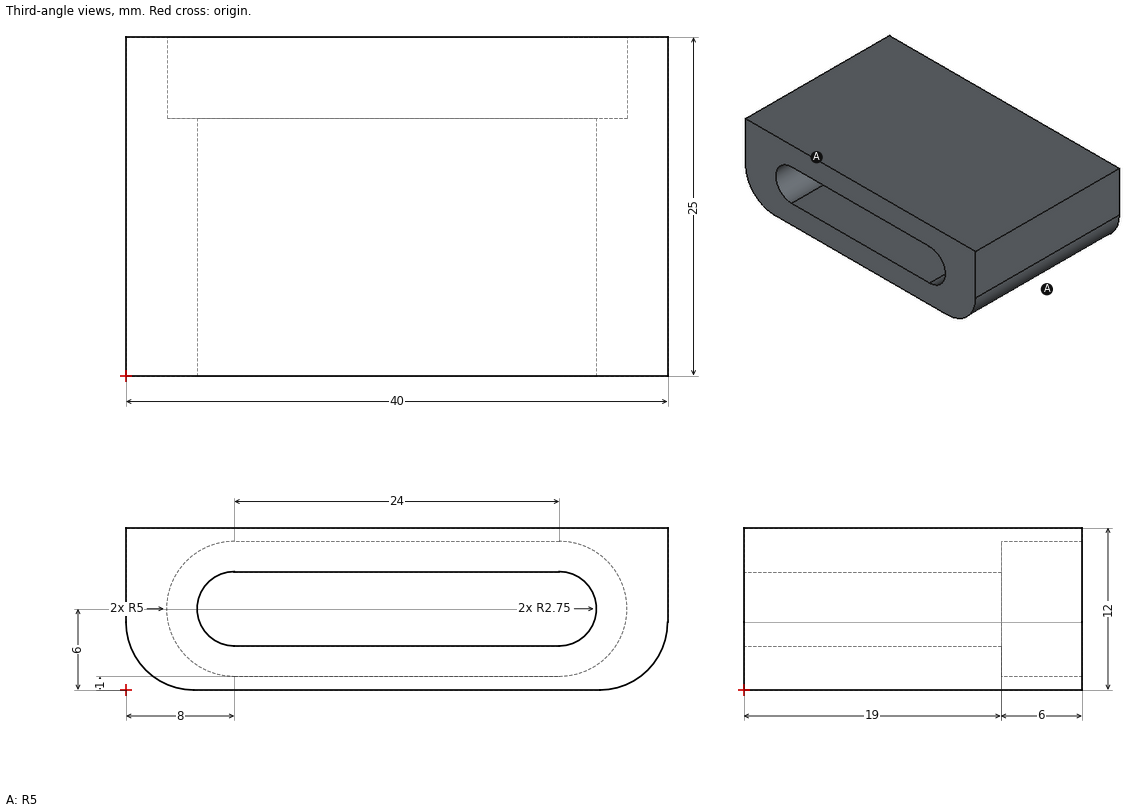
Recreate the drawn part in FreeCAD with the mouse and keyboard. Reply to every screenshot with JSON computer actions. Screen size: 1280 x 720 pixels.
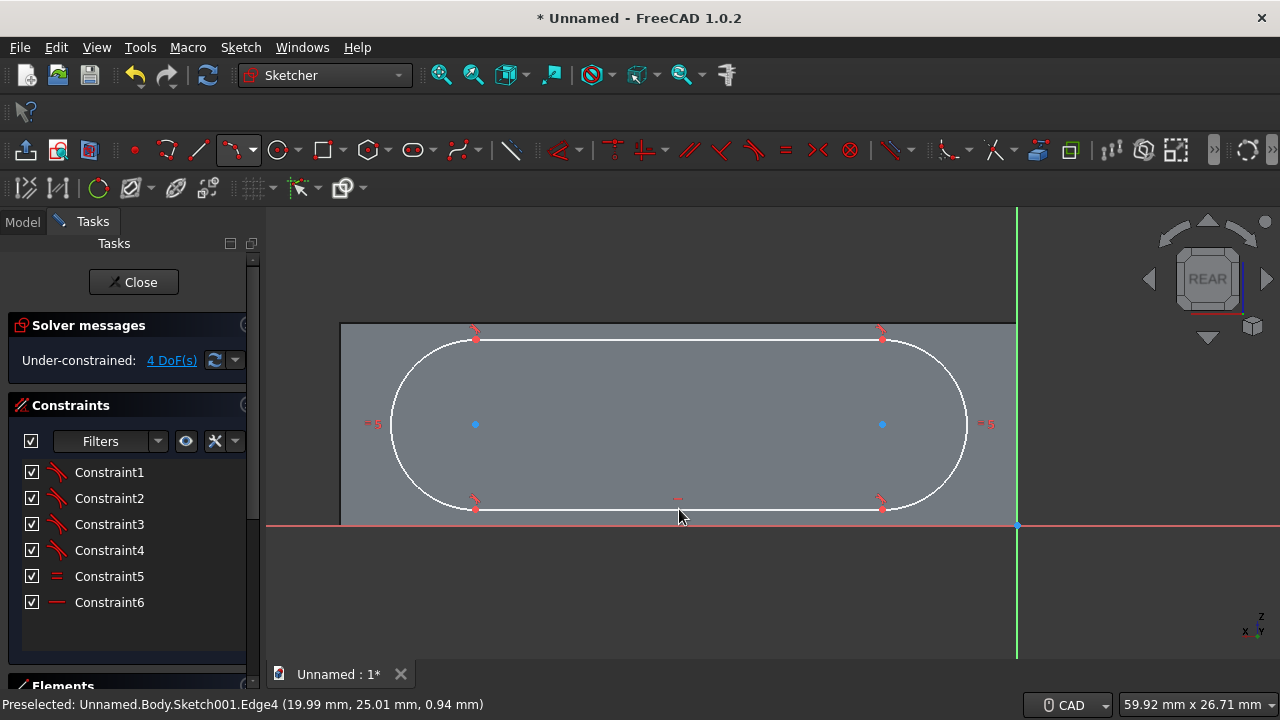
{"action": "key", "text": "d"}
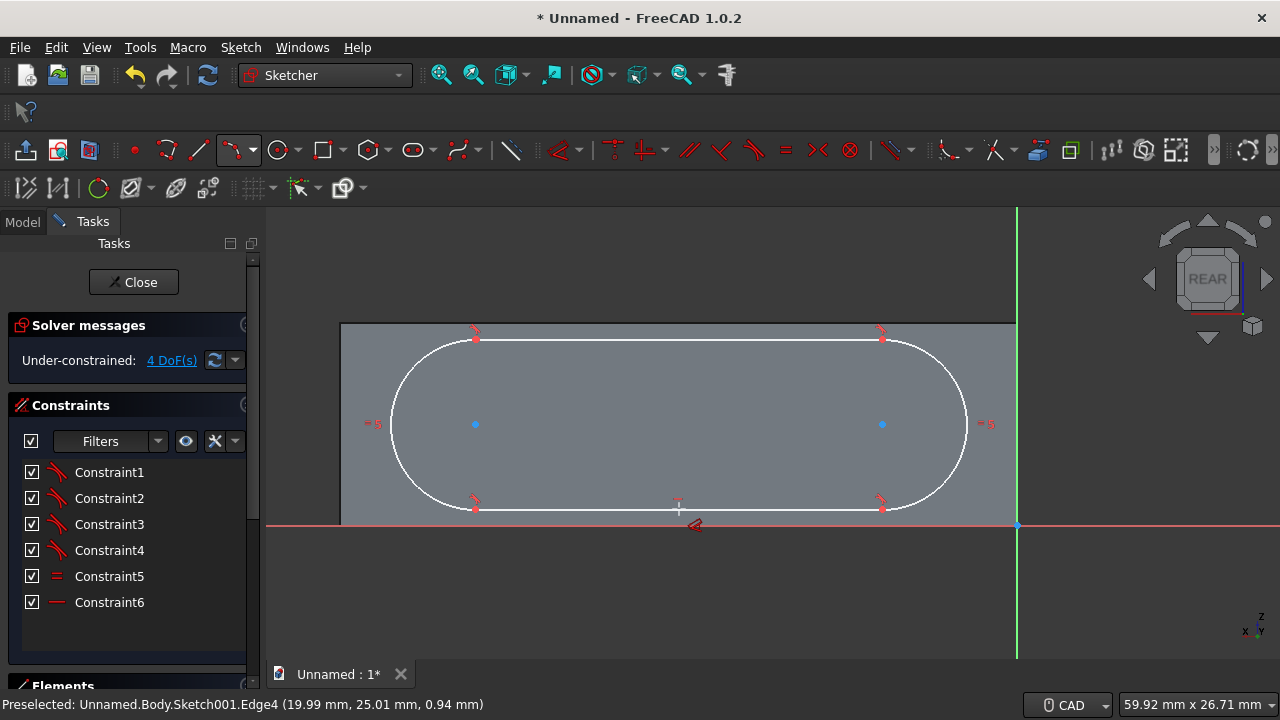
{"action": "left_click", "coordinate": [407, 375]}
{"action": "left_click", "coordinate": [381, 356]}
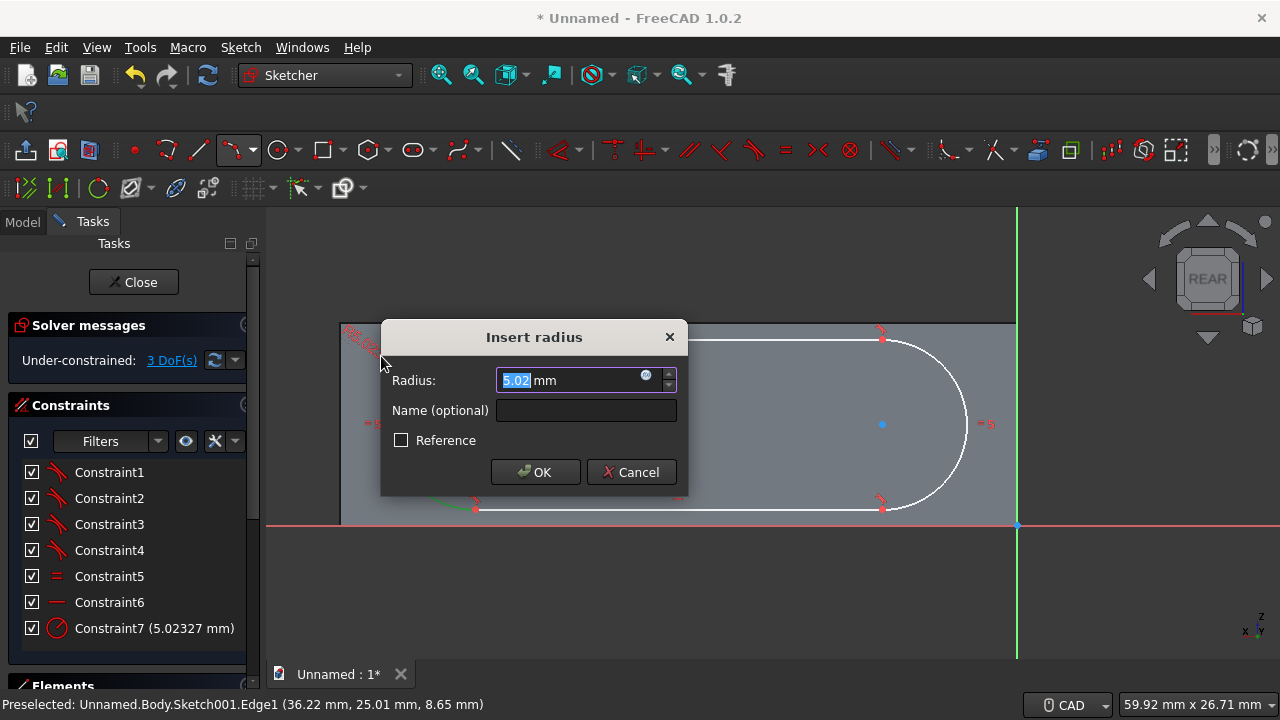
{"action": "type", "text": "5"}
{"action": "key", "text": "Return"}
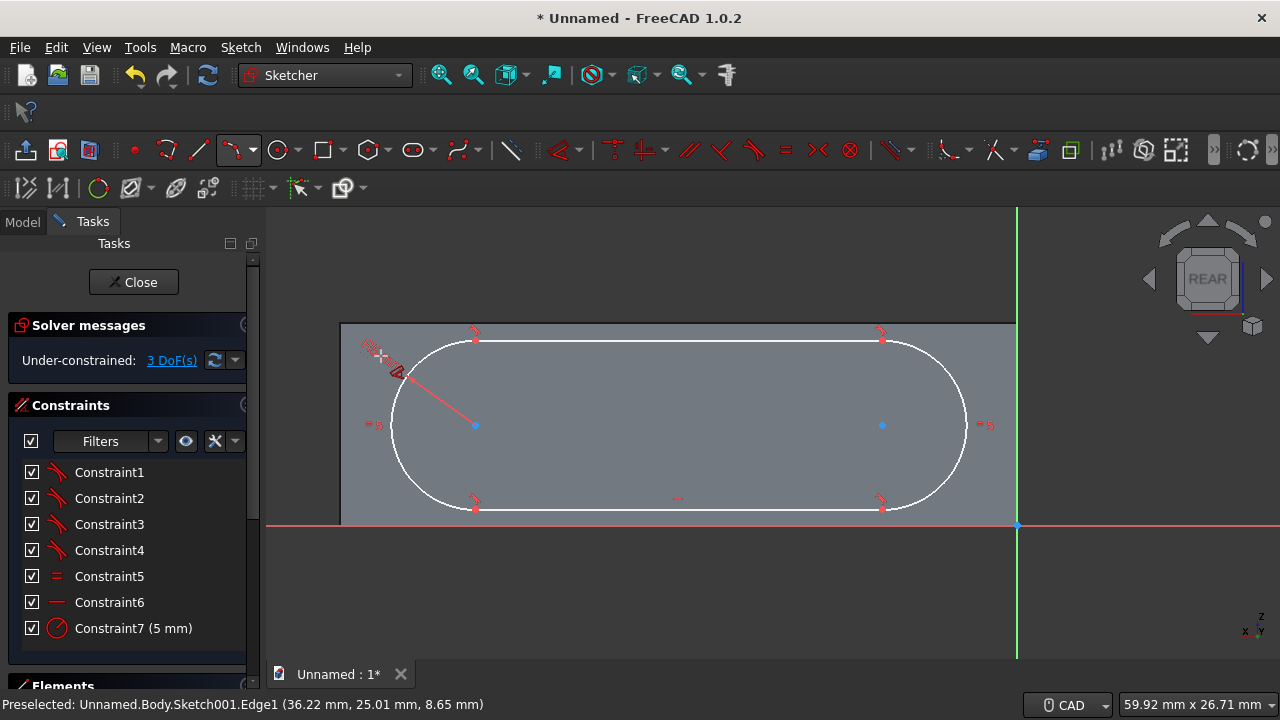
{"action": "left_click", "coordinate": [598, 341]}
{"action": "left_click", "coordinate": [679, 307]}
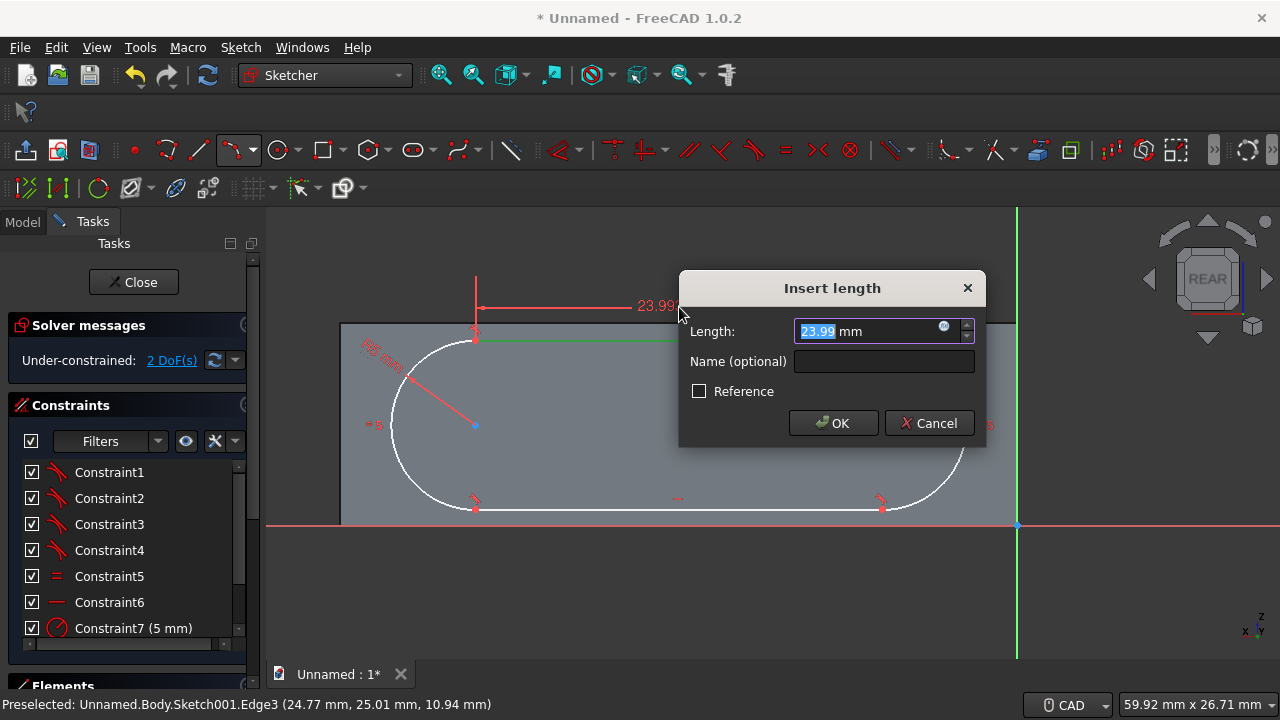
{"action": "type", "text": "24"}
{"action": "key", "text": "Return"}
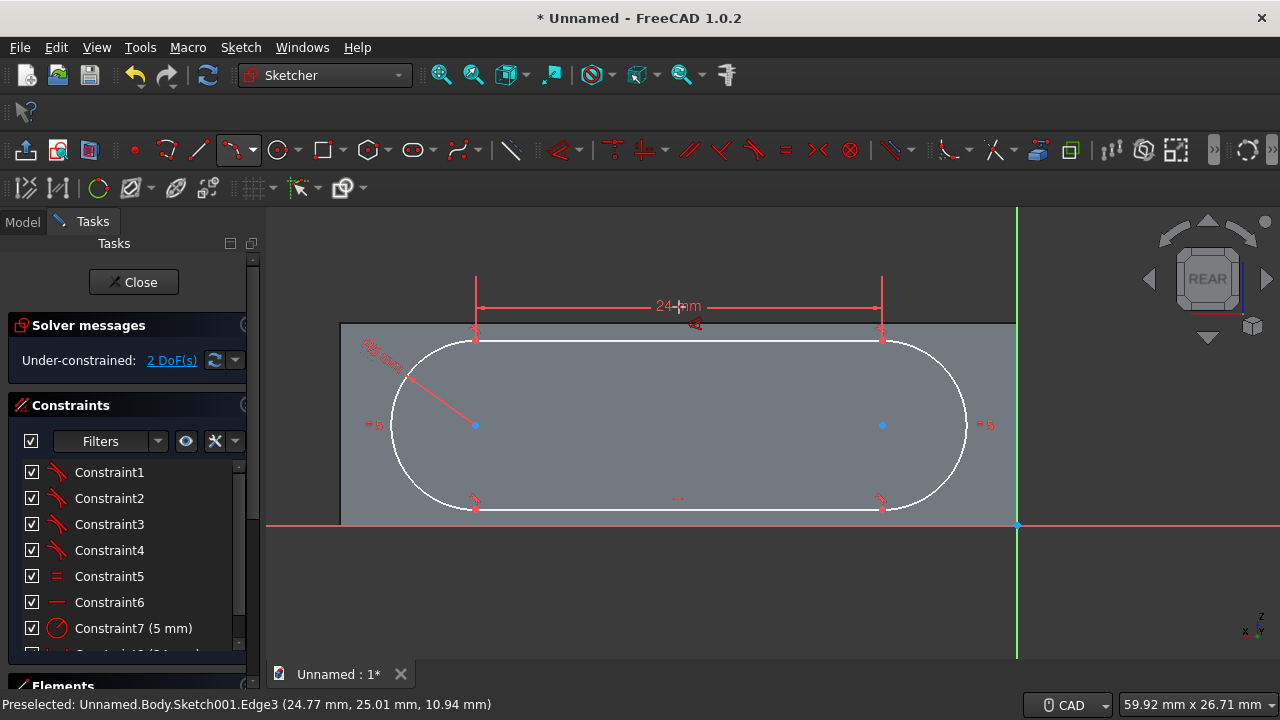
{"action": "scroll", "coordinate": [476, 510], "scroll_direction": "up", "scroll_amount": 5}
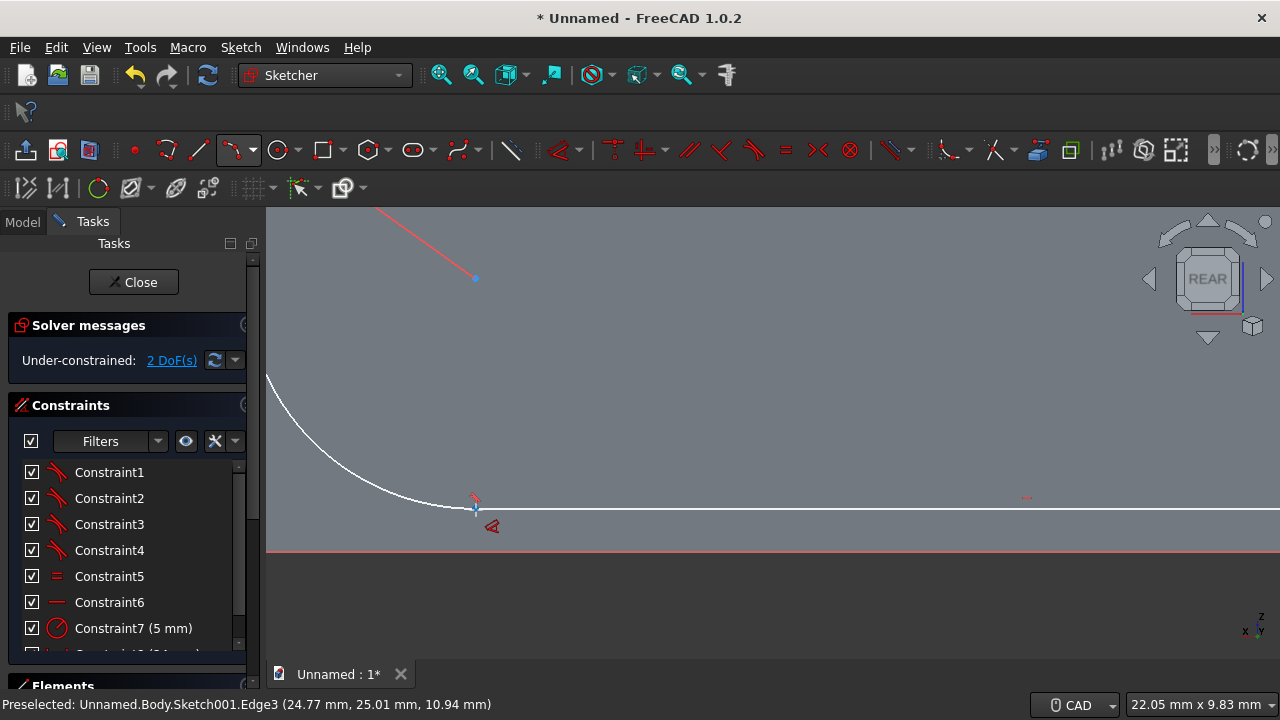
{"action": "left_click", "coordinate": [475, 509]}
{"action": "left_click", "coordinate": [441, 530]}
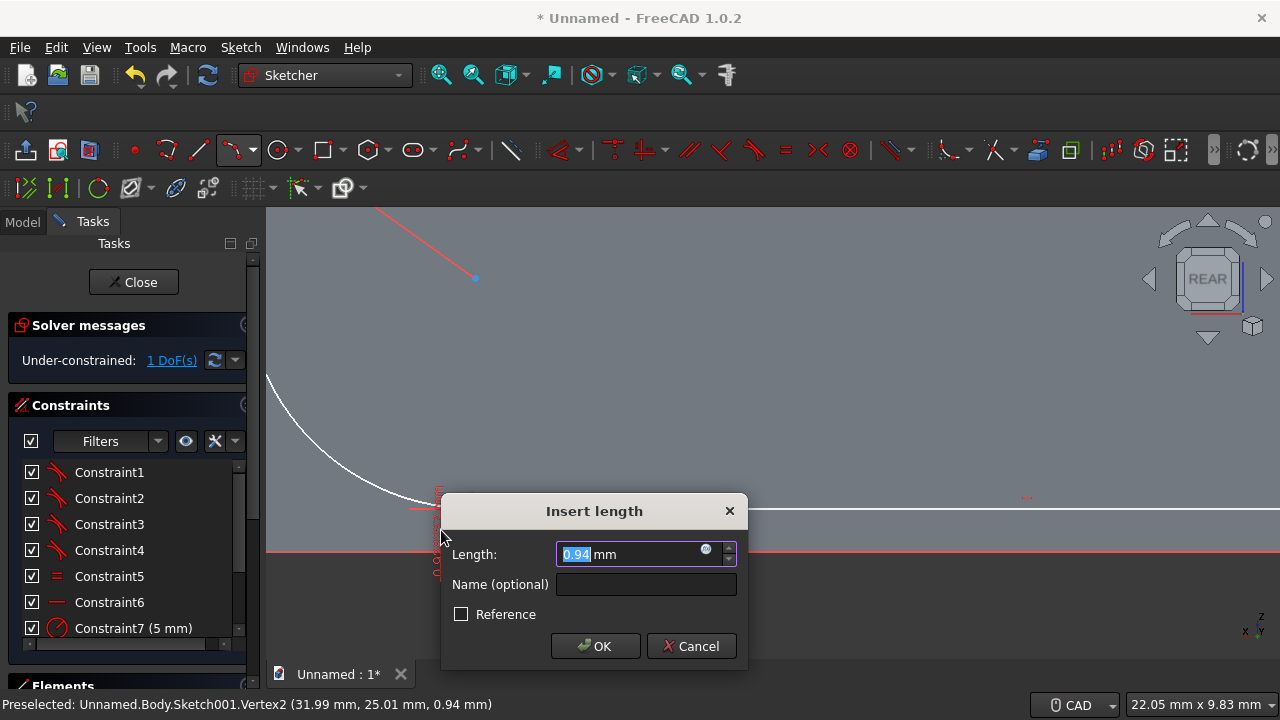
{"action": "type", "text": "1"}
{"action": "key", "text": "Return"}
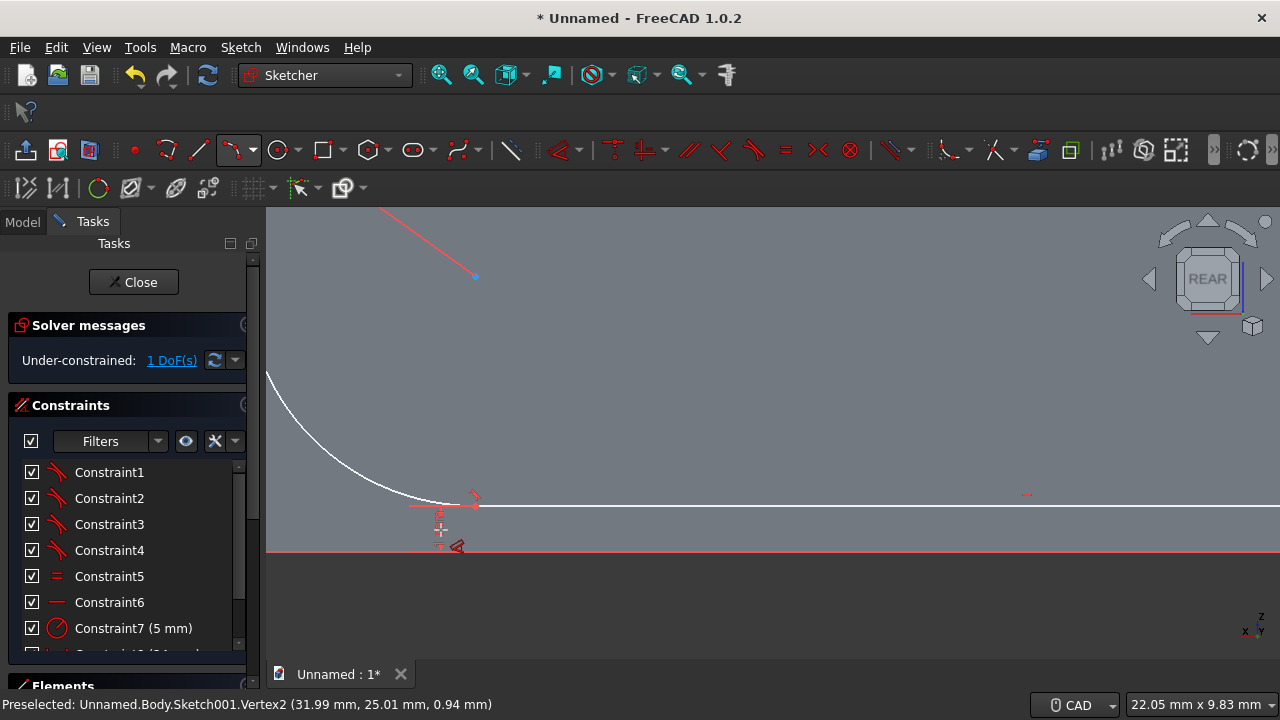
{"action": "scroll", "coordinate": [477, 511], "scroll_direction": "down", "scroll_amount": 5}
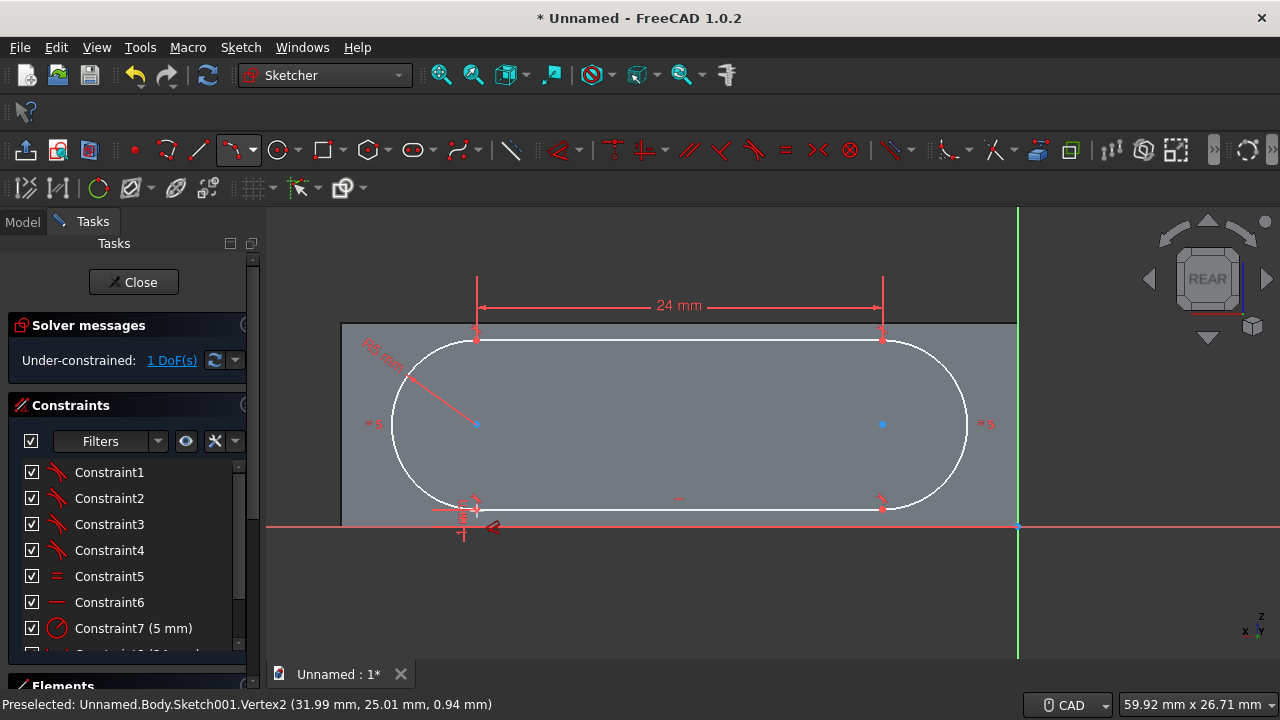
{"action": "left_click", "coordinate": [883, 510]}
{"action": "left_click", "coordinate": [950, 561]}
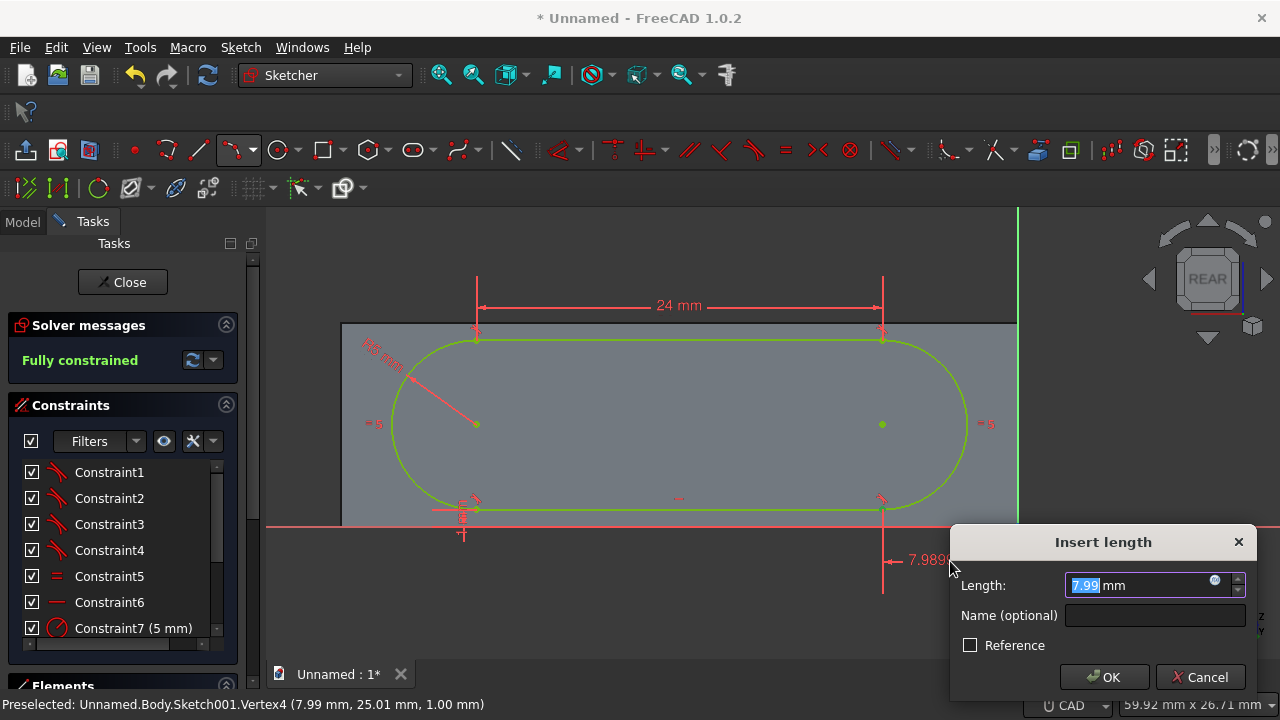
{"action": "type", "text": "8"}
{"action": "key", "text": "Return"}
{"action": "key", "text": "Escape"}